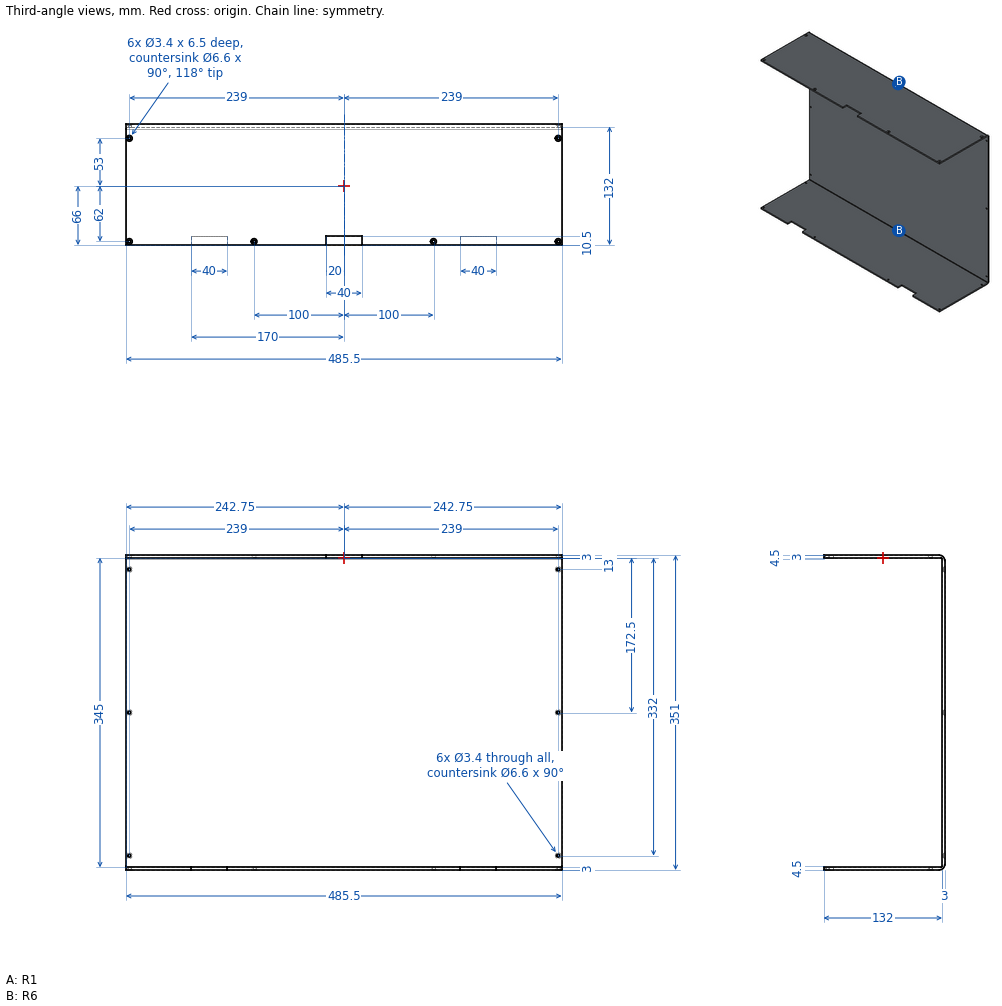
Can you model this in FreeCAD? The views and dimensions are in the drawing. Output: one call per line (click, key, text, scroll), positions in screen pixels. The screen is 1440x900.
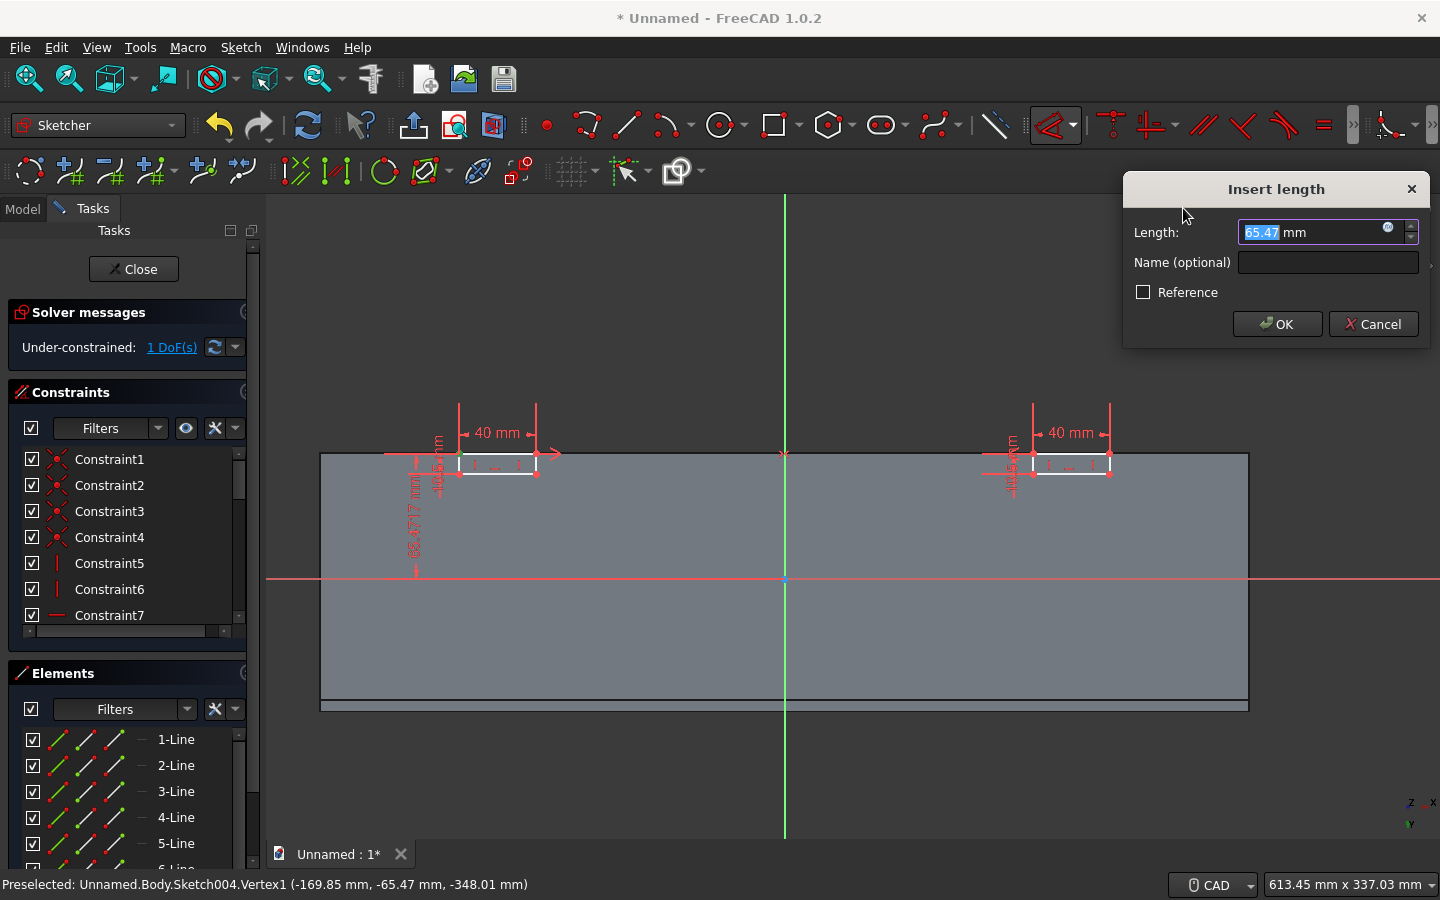
text(66)
key(Return)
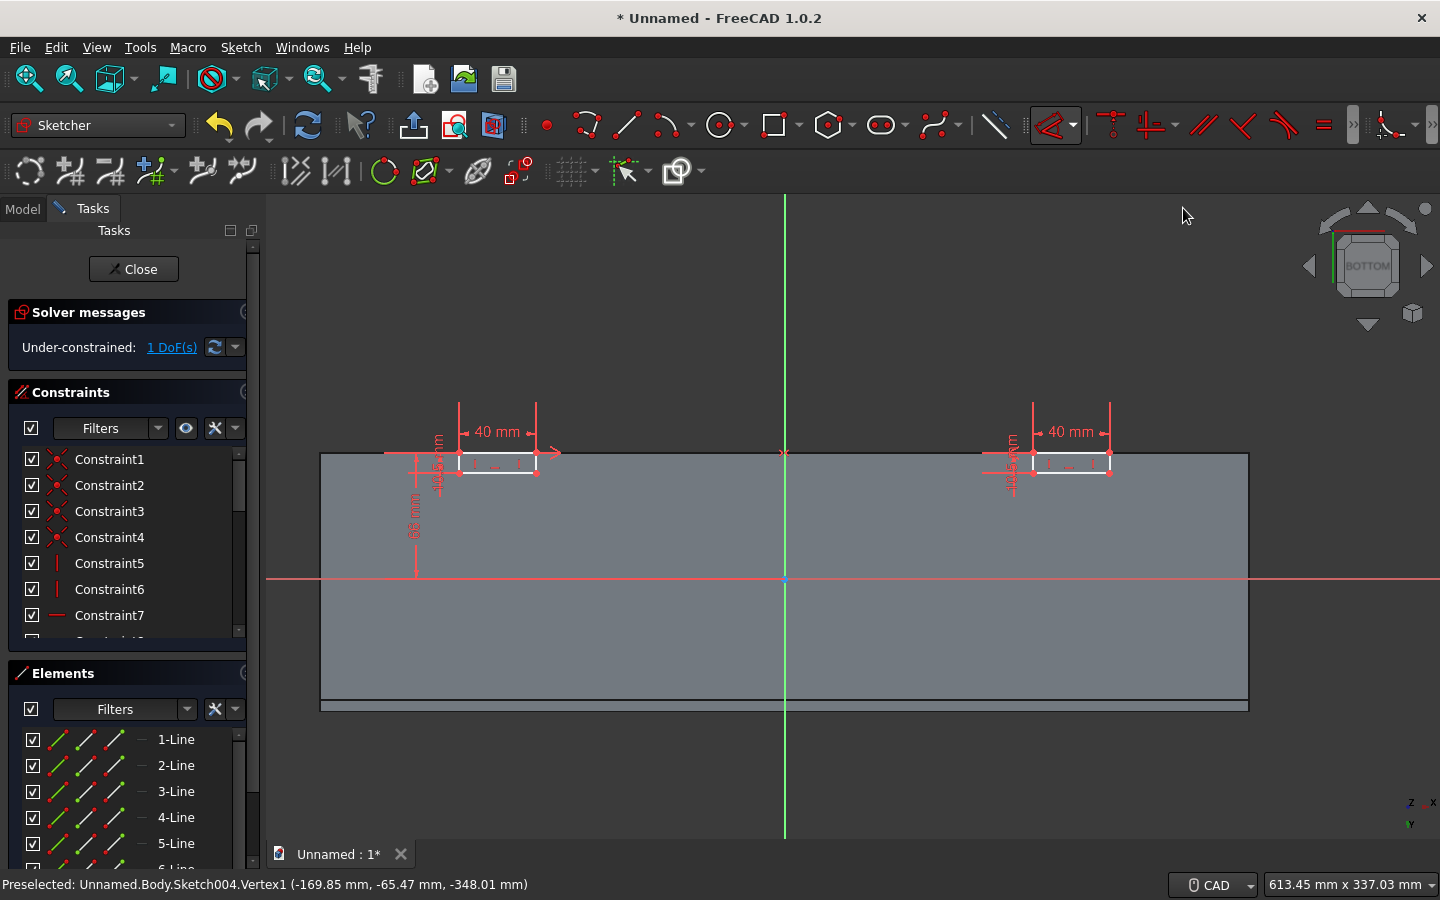
click(459, 453)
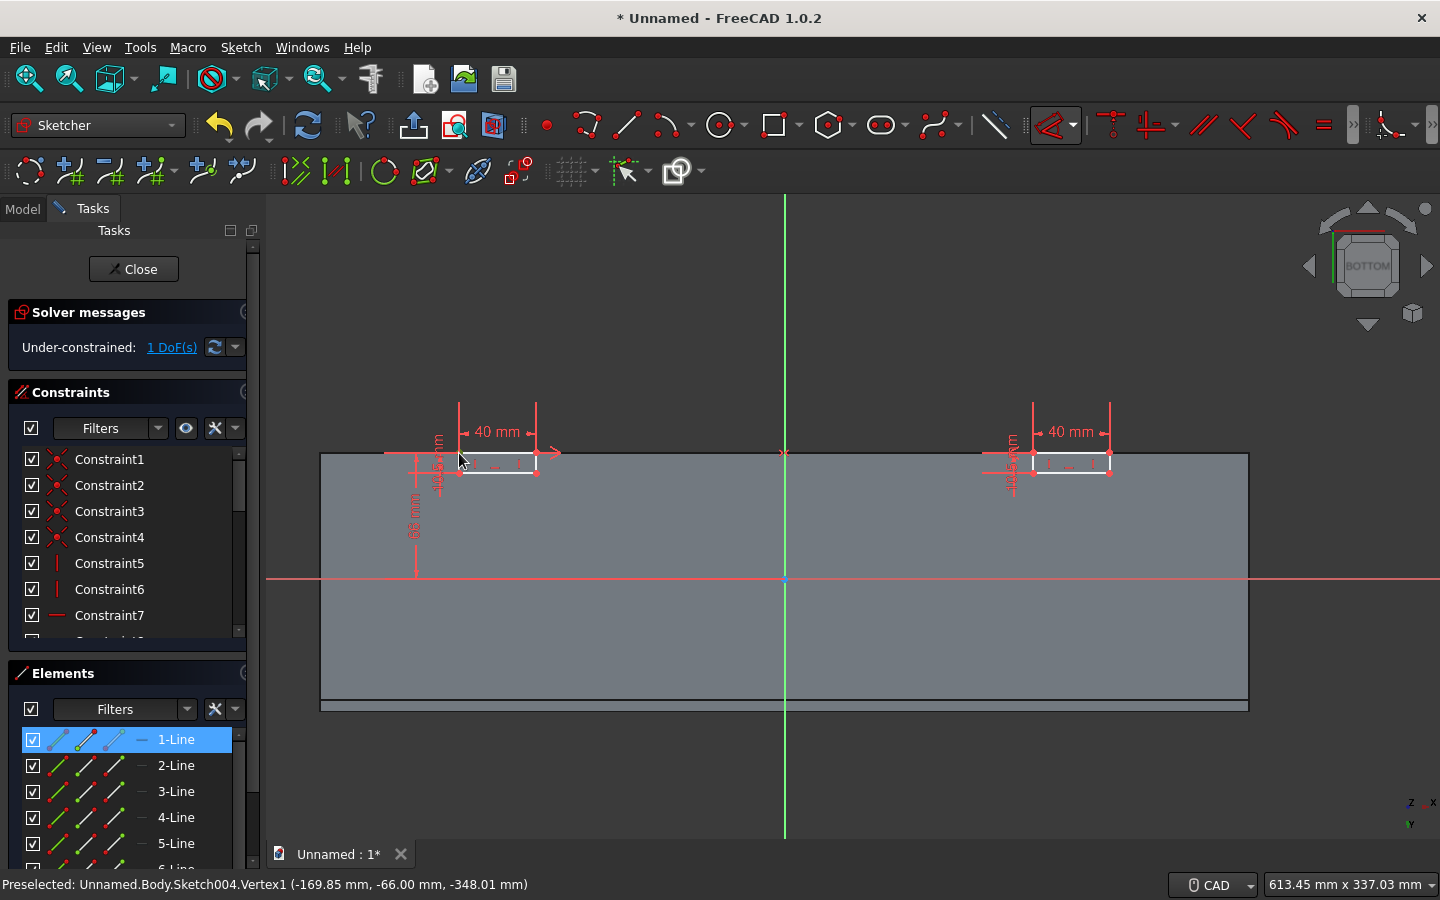
key(l)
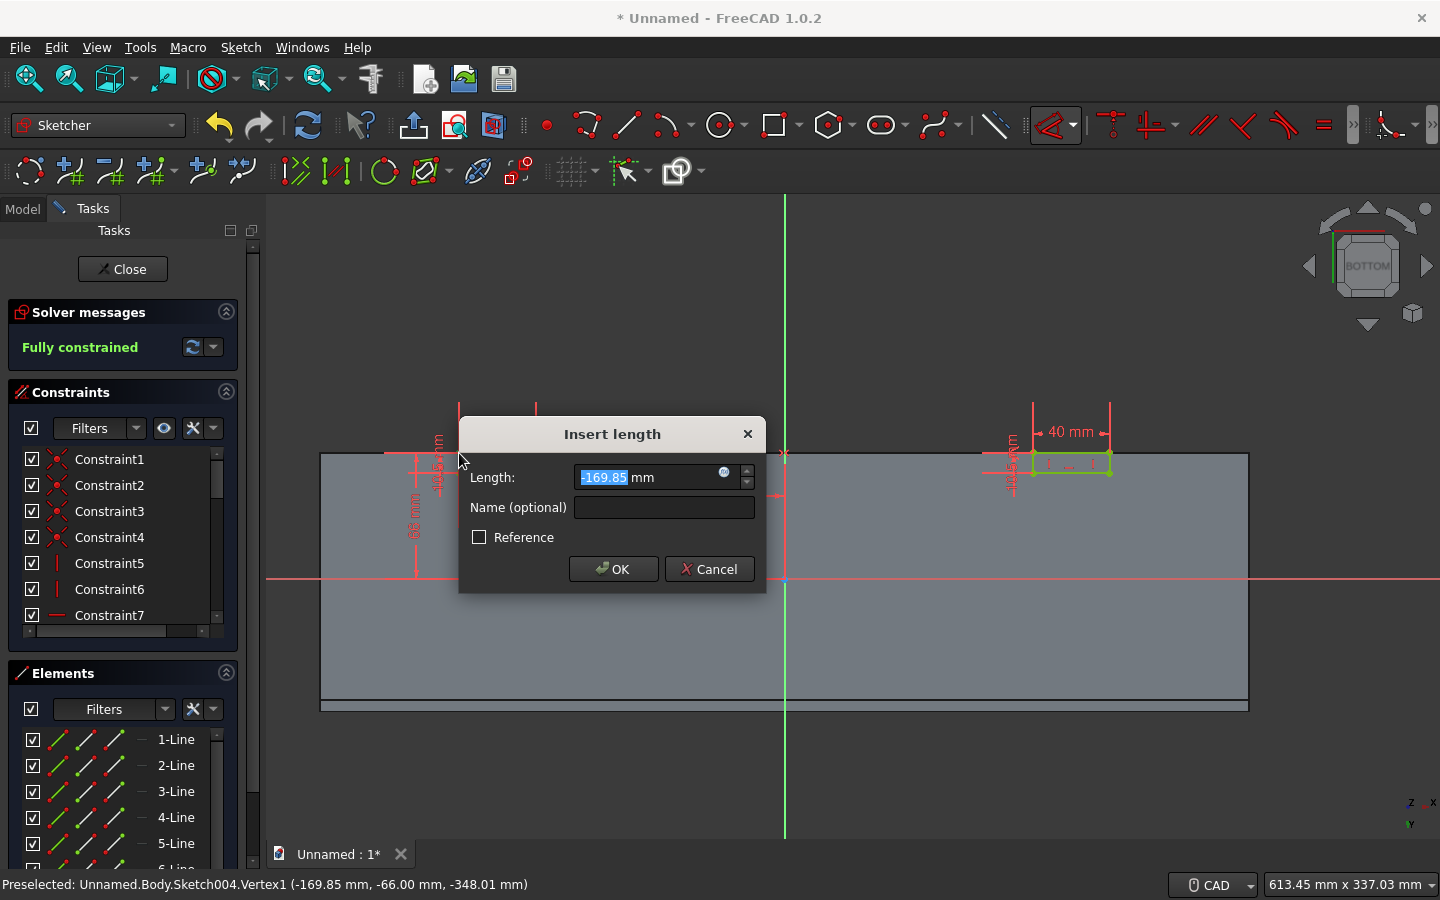
text(-170)
key(Return)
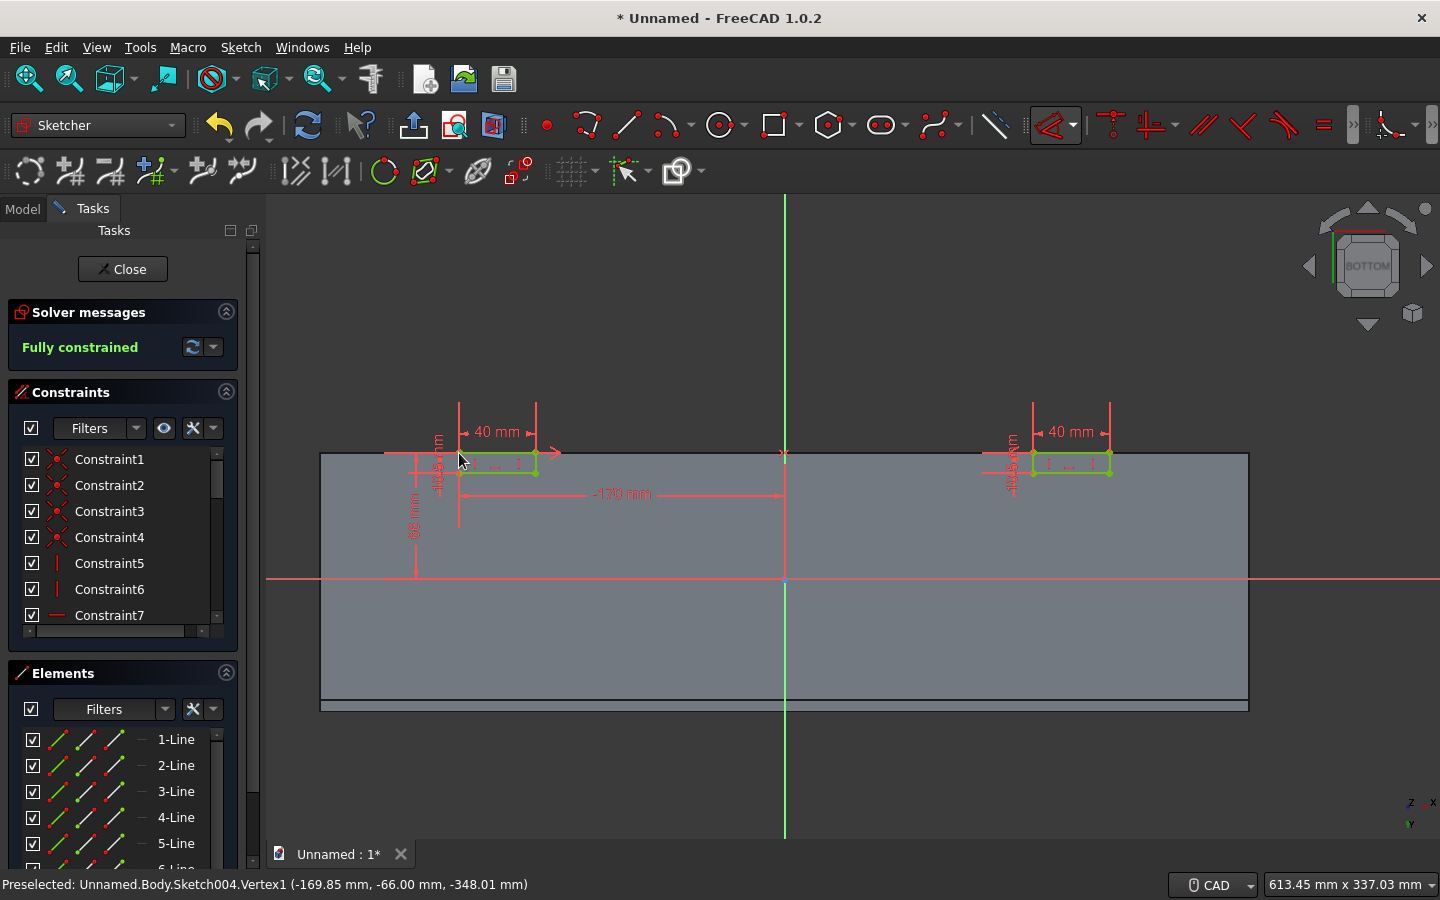
click(123, 269)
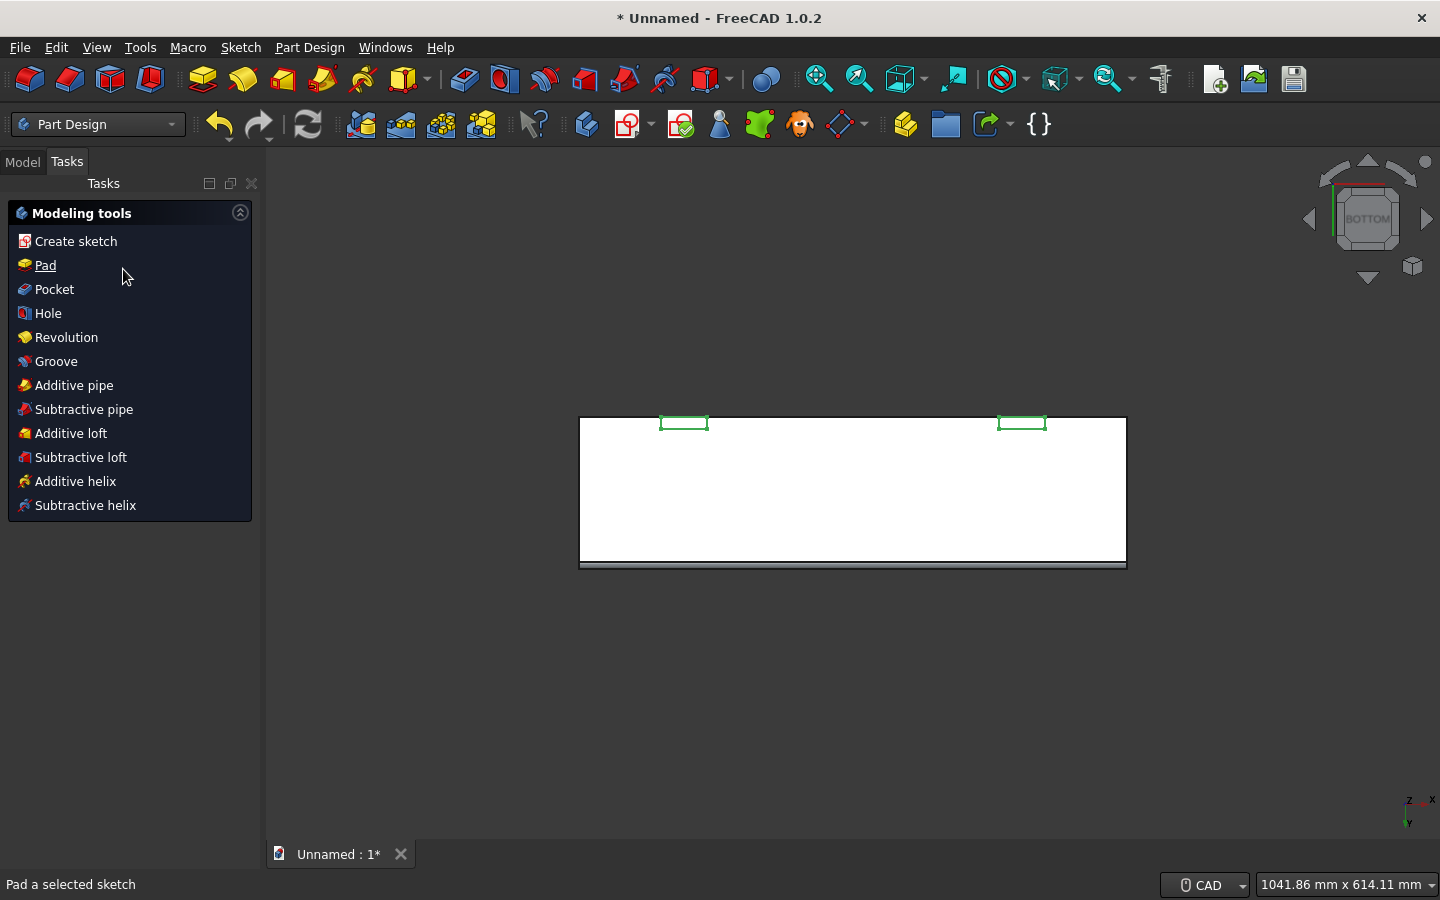
click(466, 80)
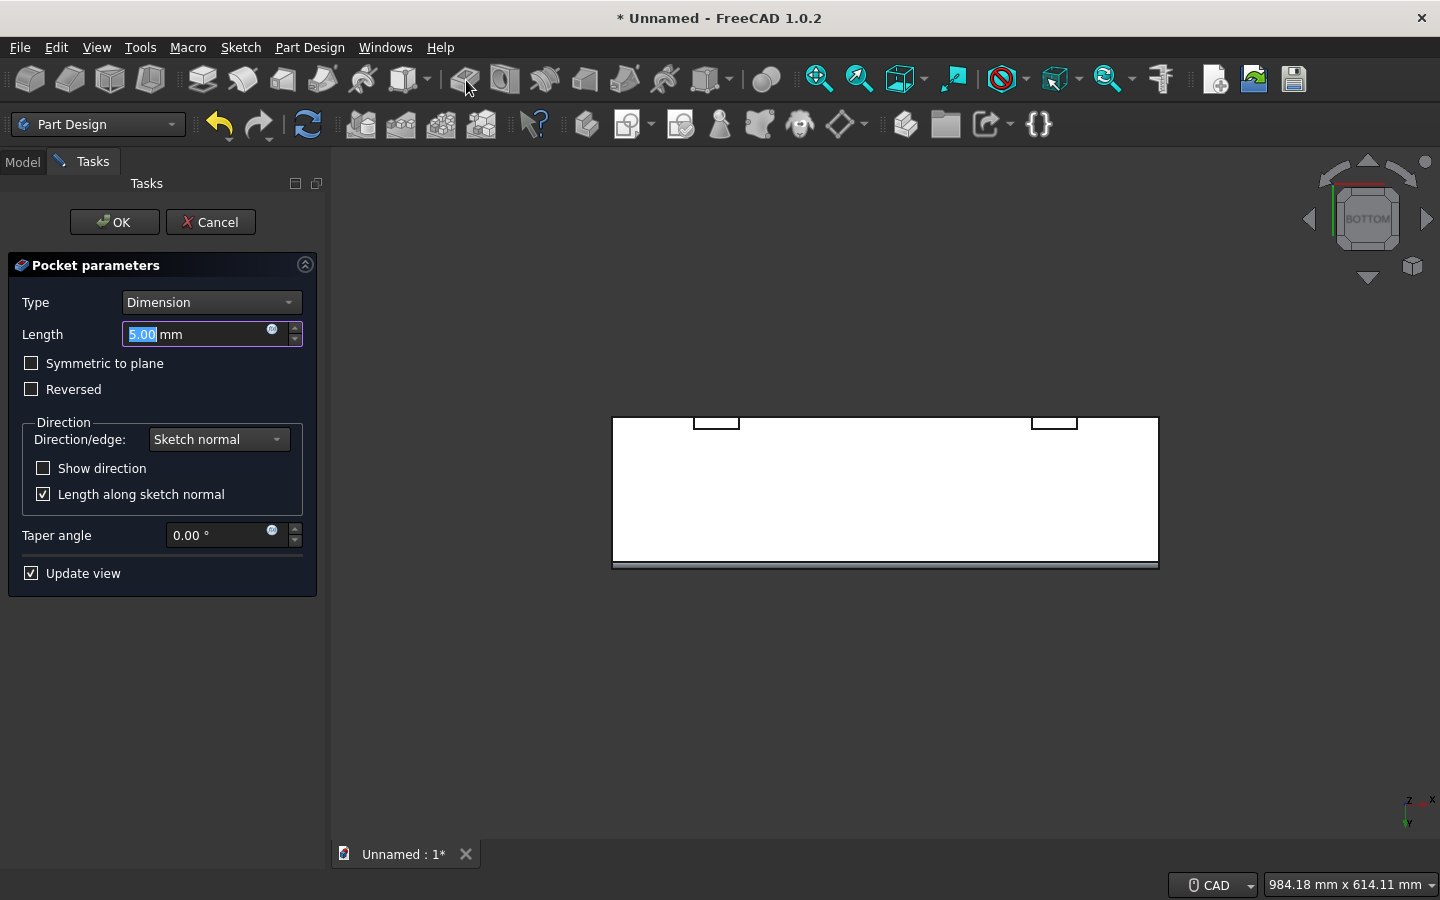
text(4.5)
key(Tab)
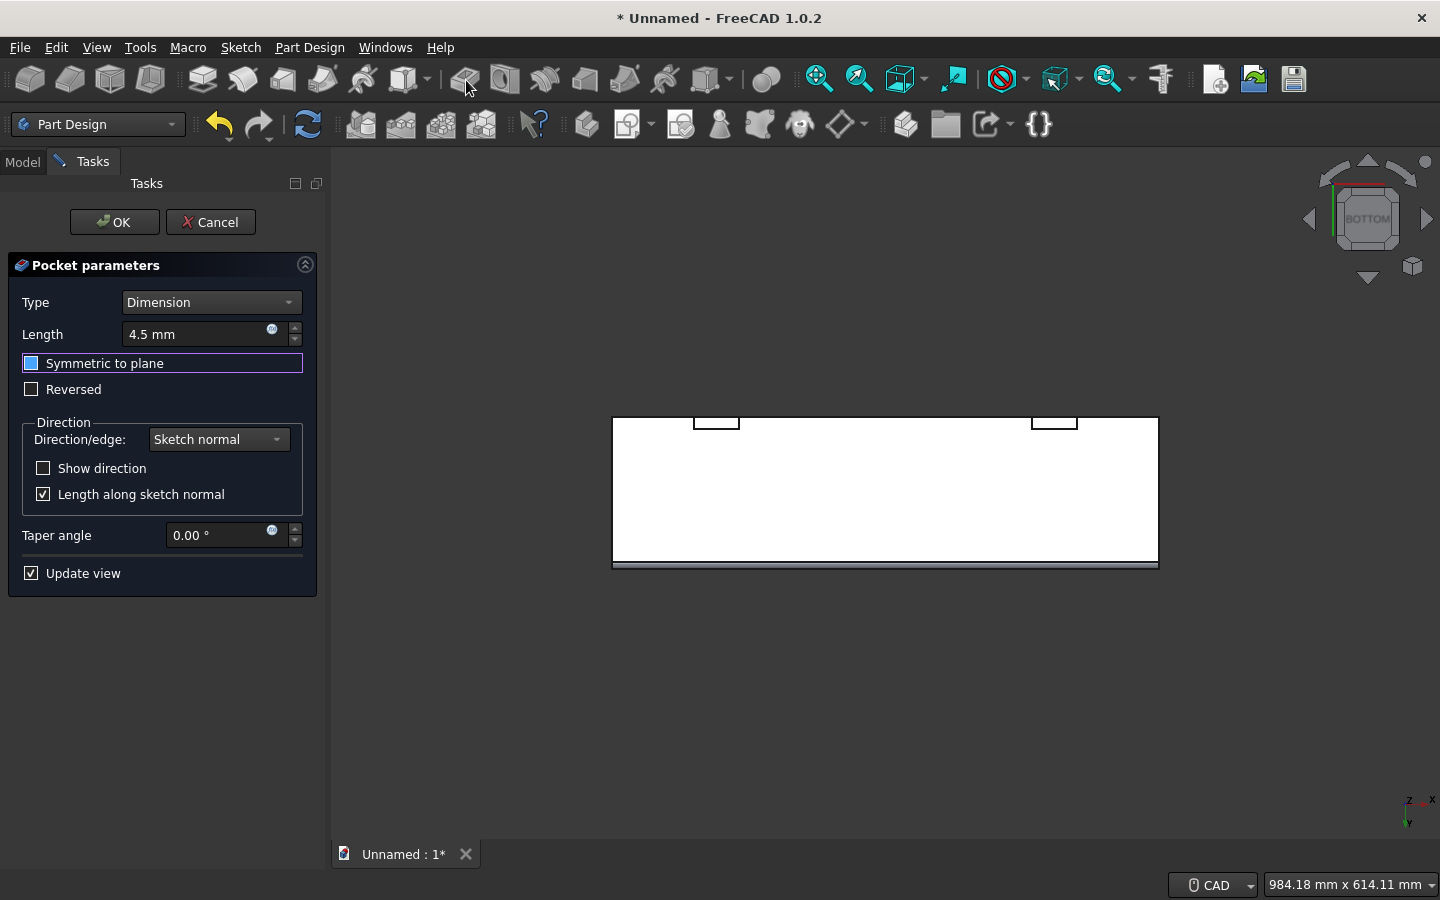
click(115, 222)